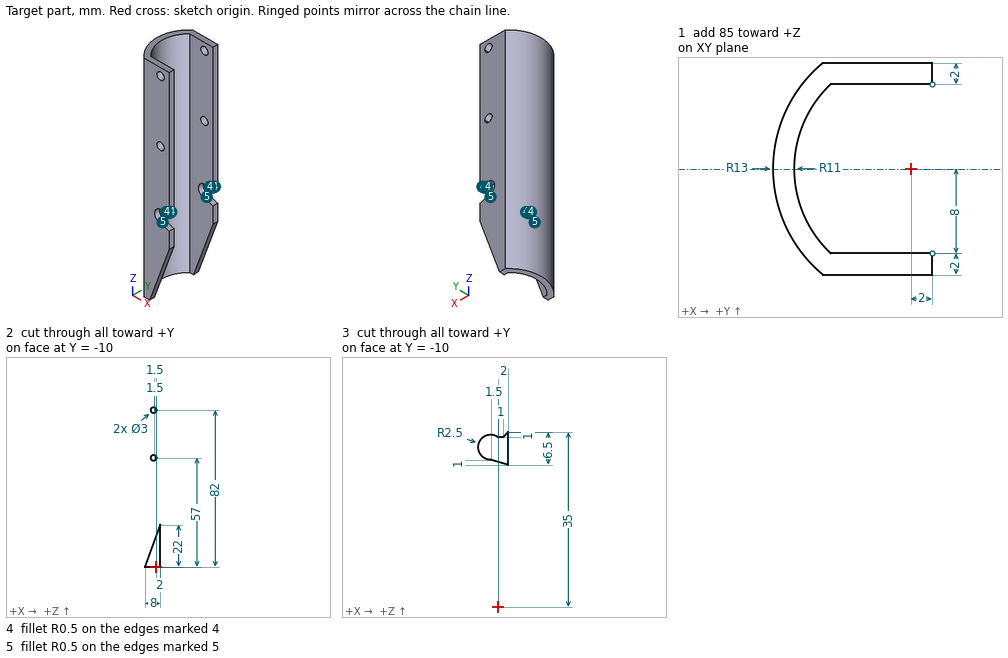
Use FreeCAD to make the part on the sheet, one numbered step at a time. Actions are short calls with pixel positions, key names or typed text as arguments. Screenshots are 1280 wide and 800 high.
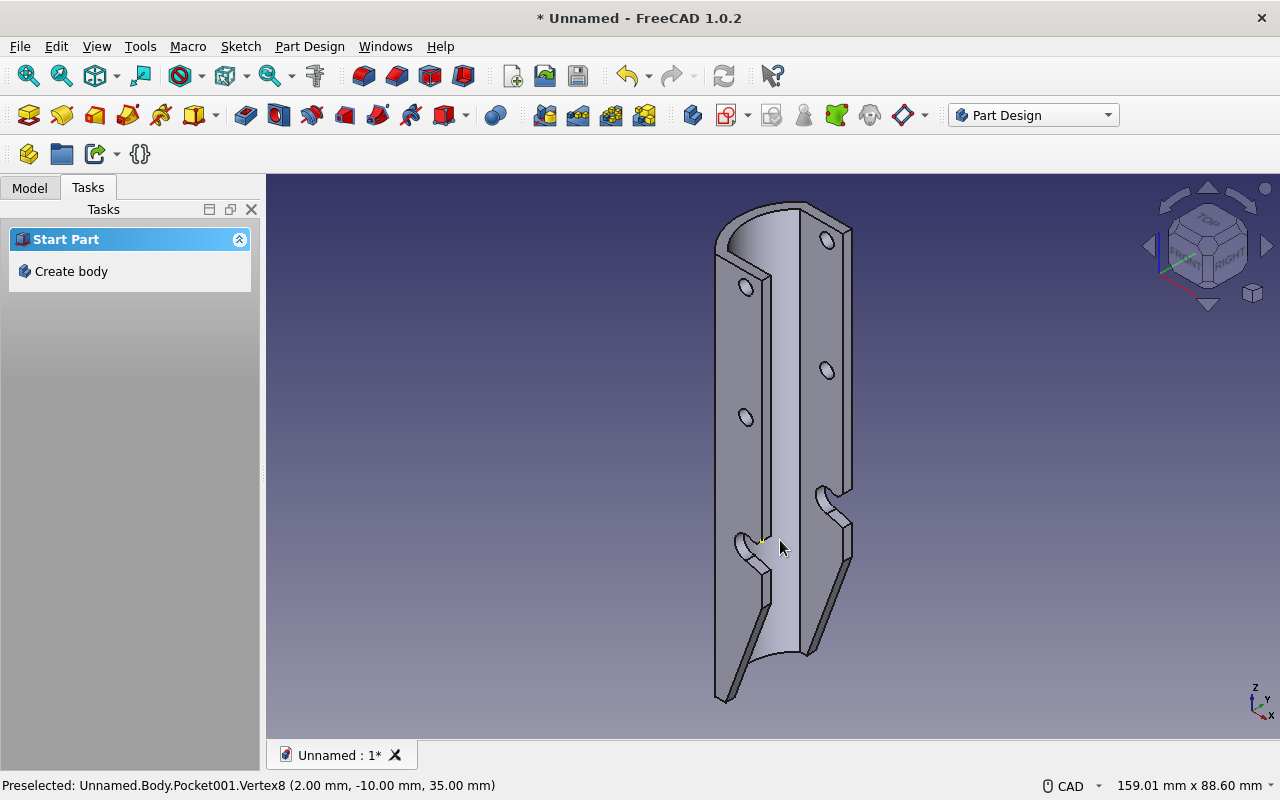
scroll(762, 540, up, 6)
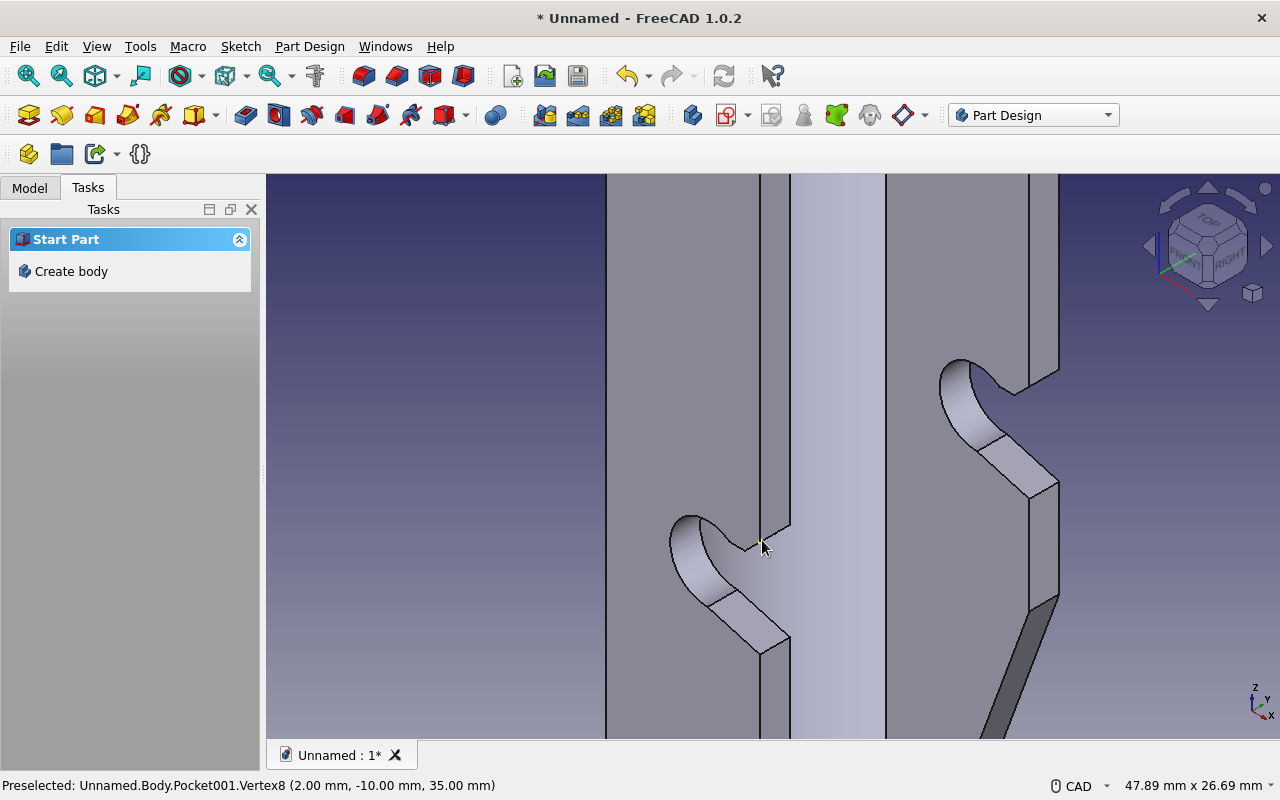
click(29, 76)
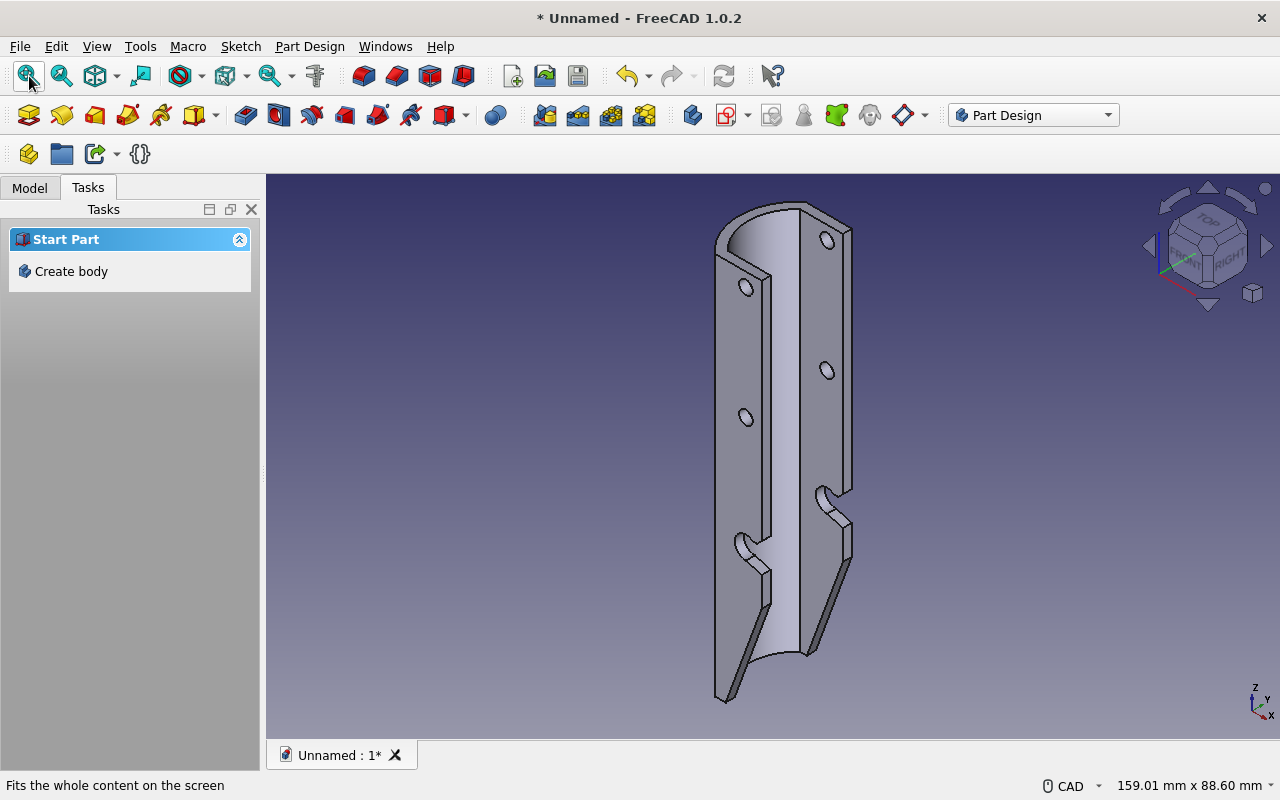
key(2)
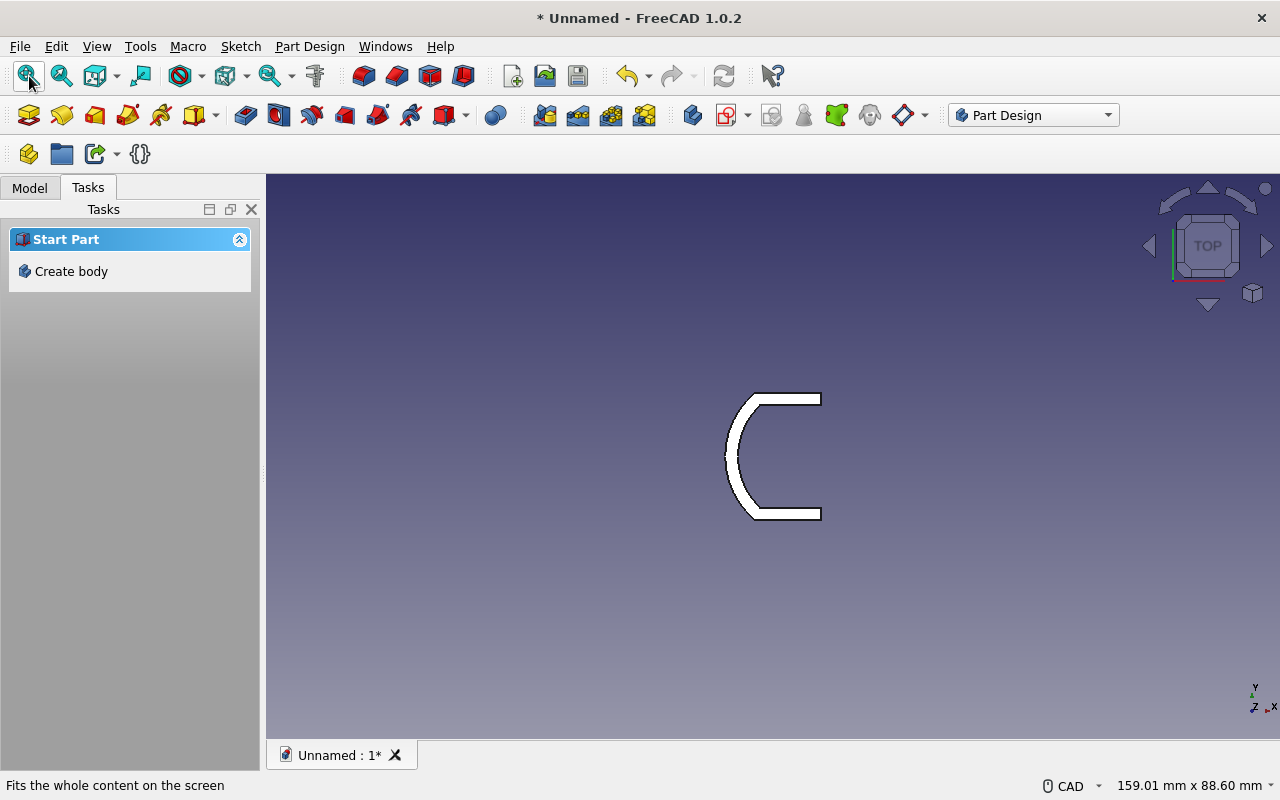
key(v)
key(f)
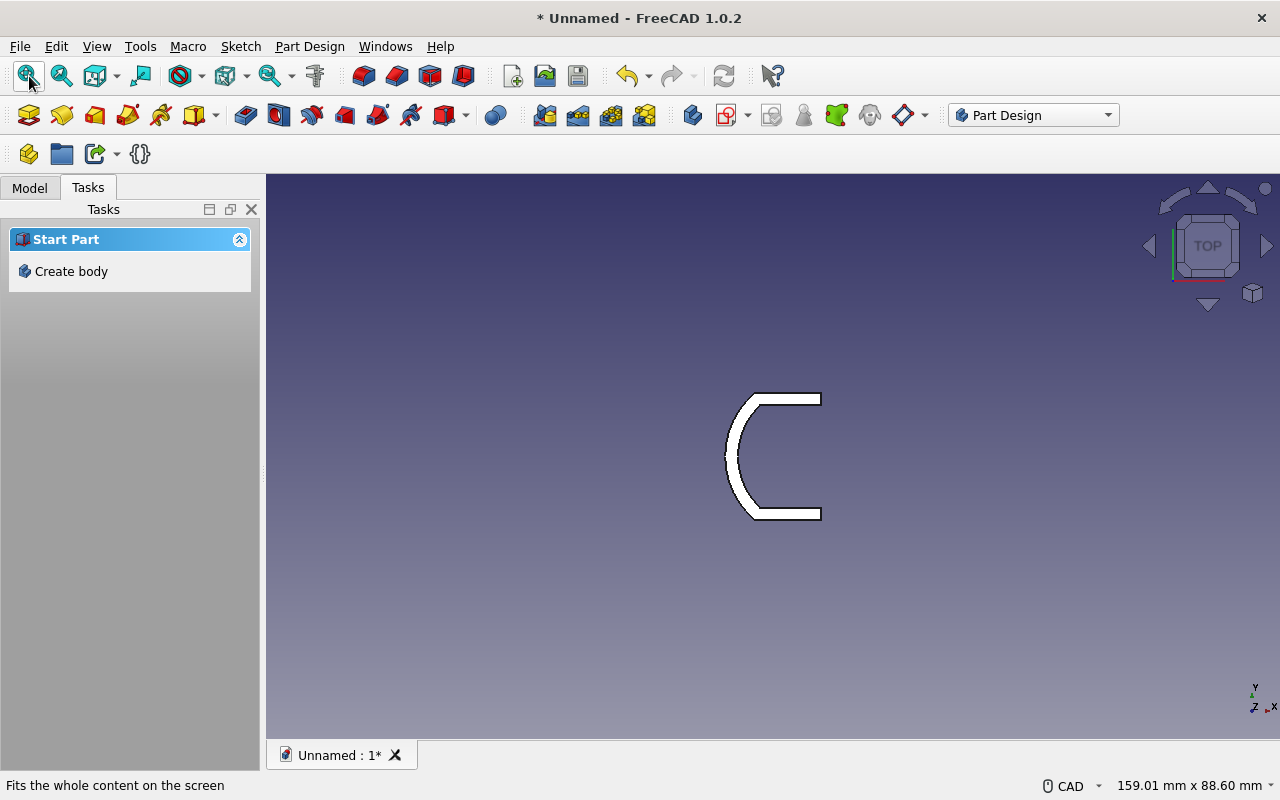
scroll(814, 513, up, 6)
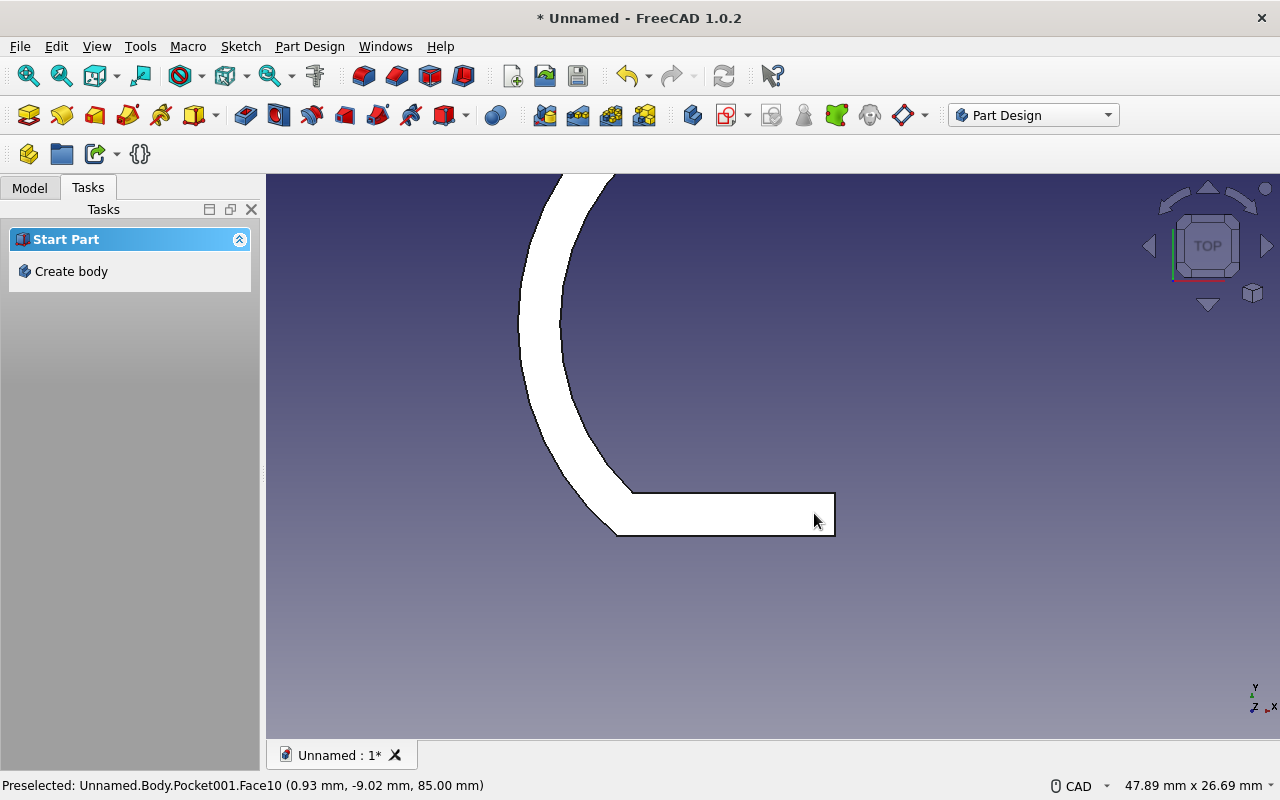
key(v)
key(f)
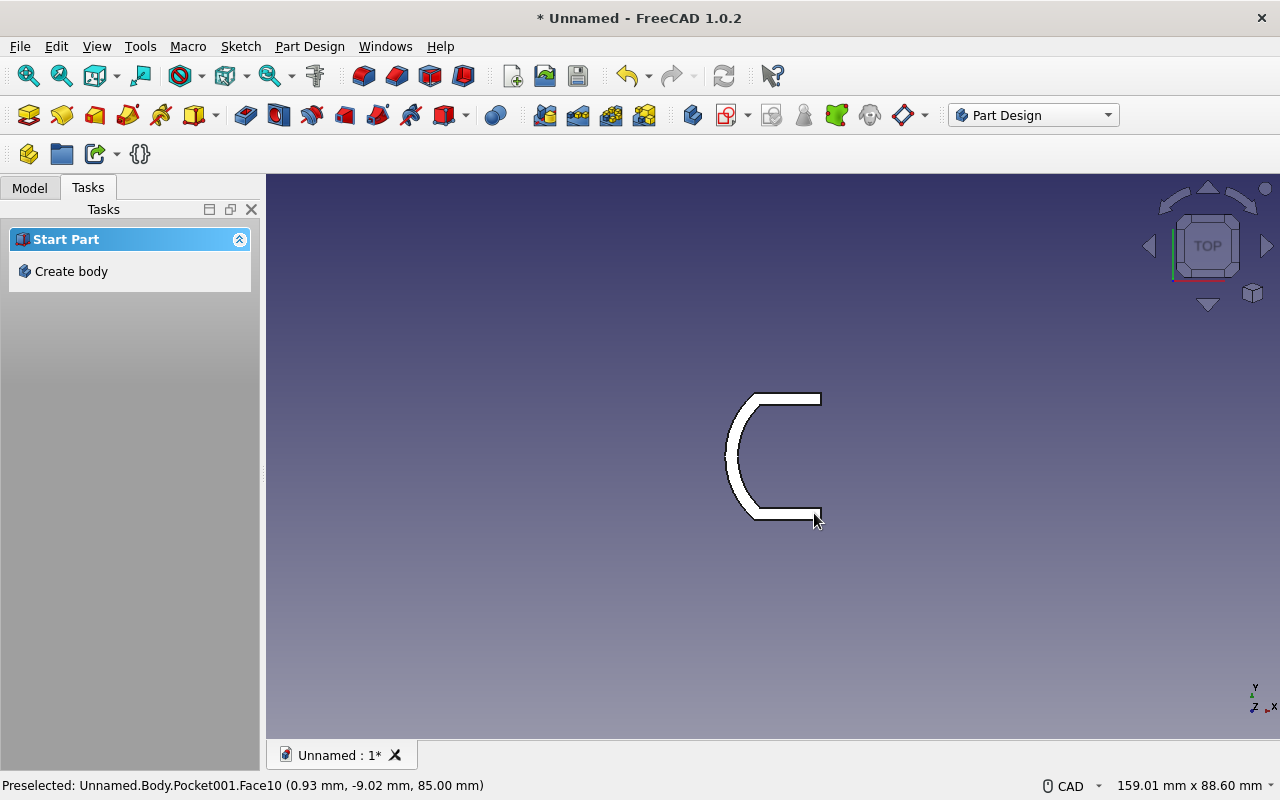
key(1)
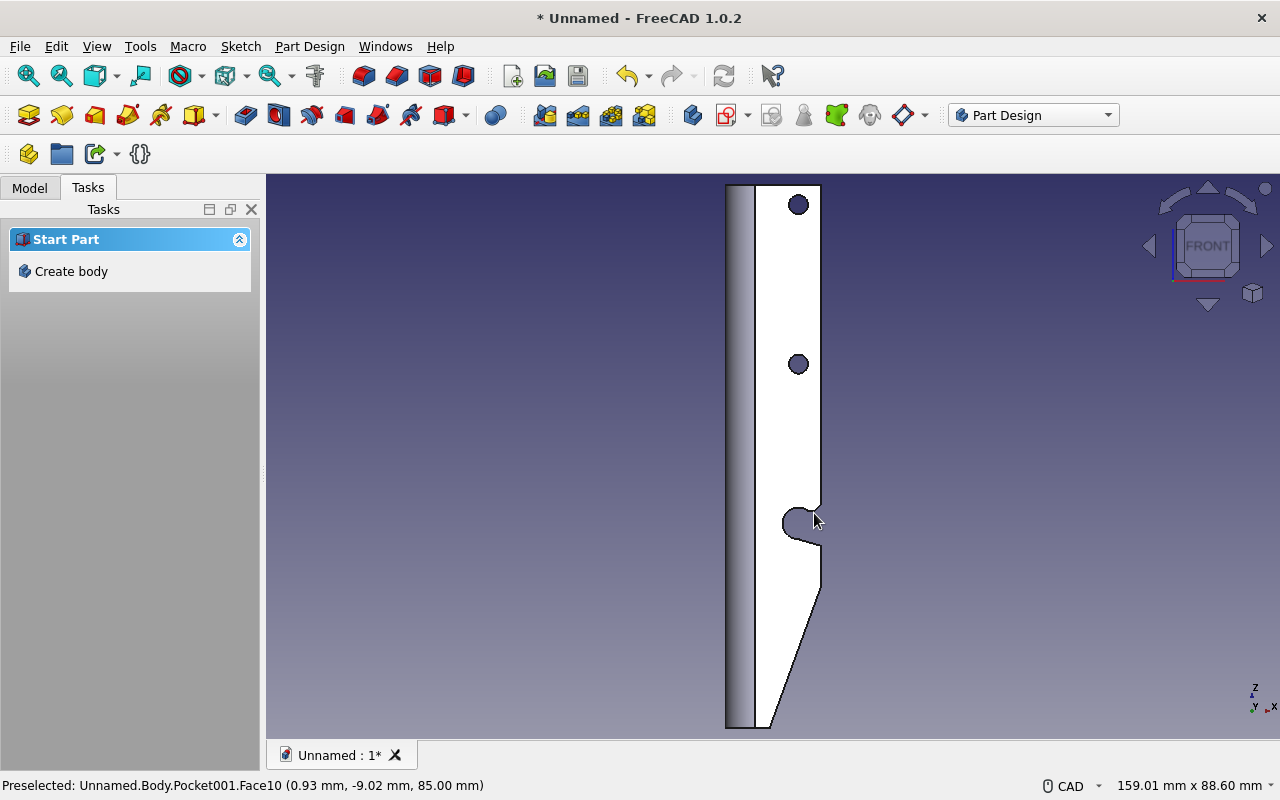
scroll(814, 510, up, 6)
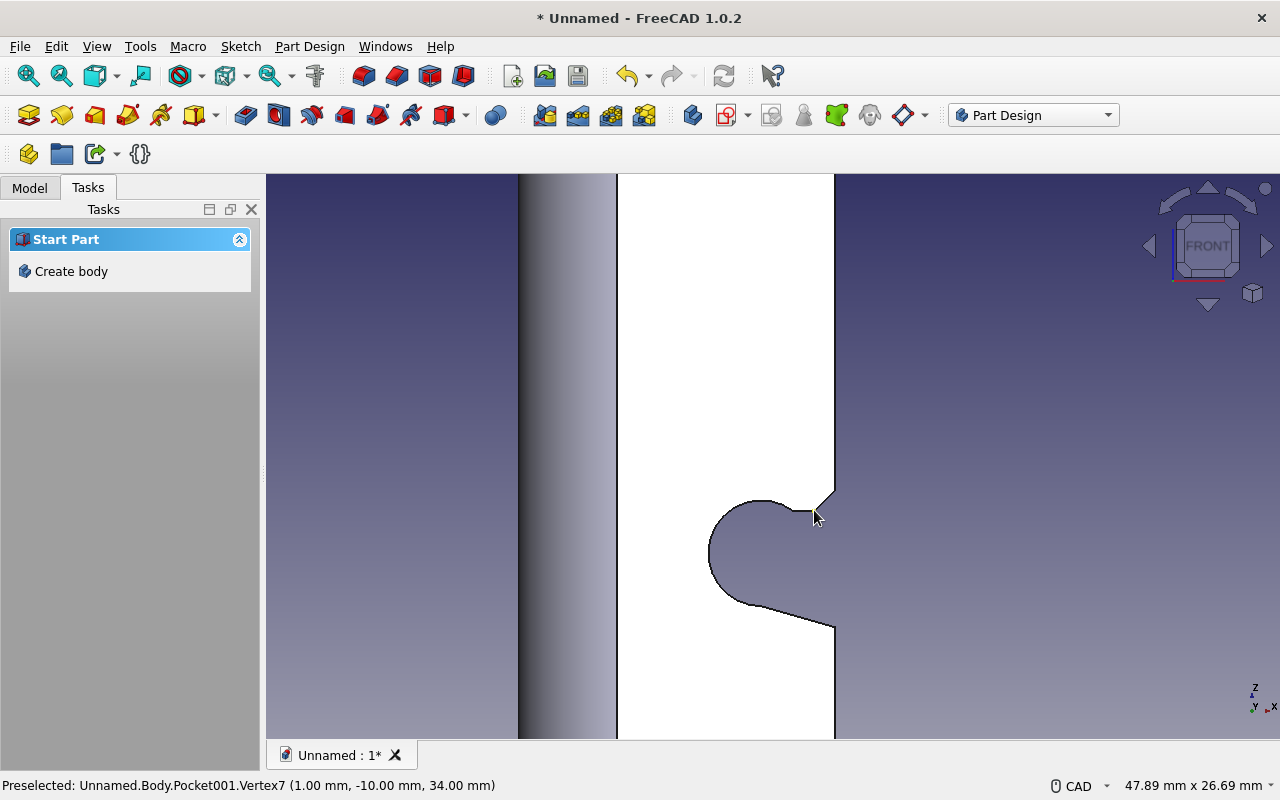
click(29, 76)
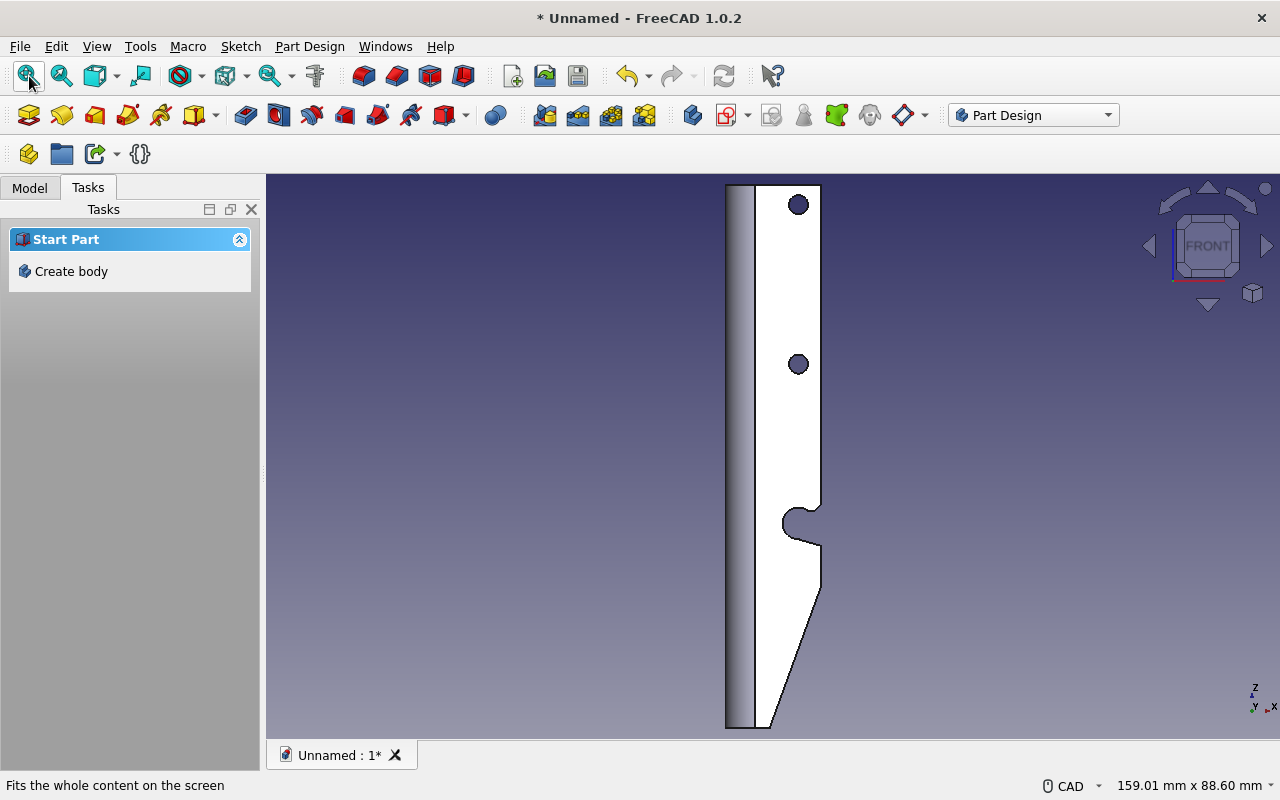
key(3)